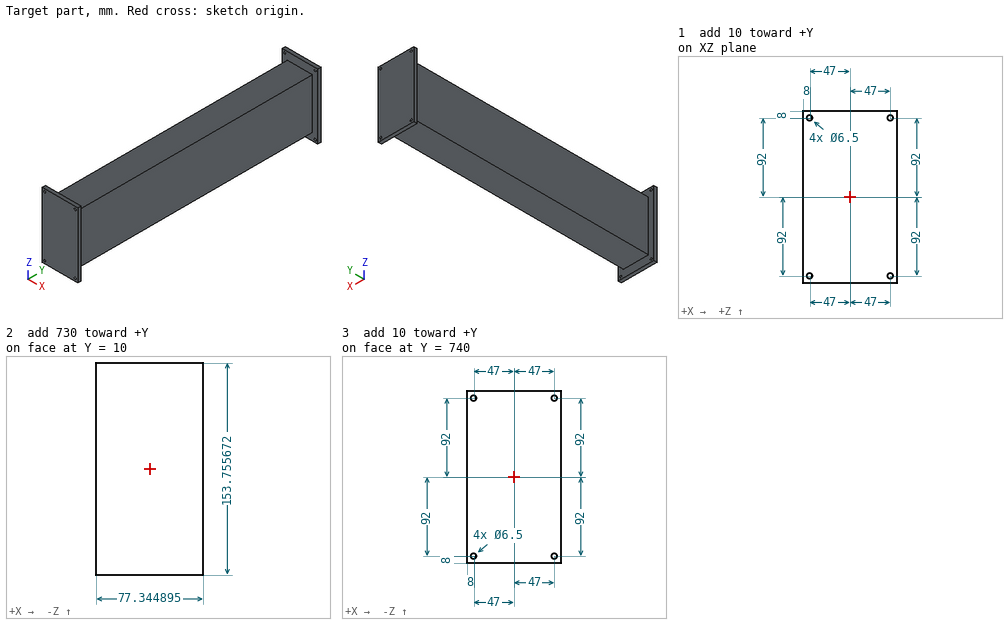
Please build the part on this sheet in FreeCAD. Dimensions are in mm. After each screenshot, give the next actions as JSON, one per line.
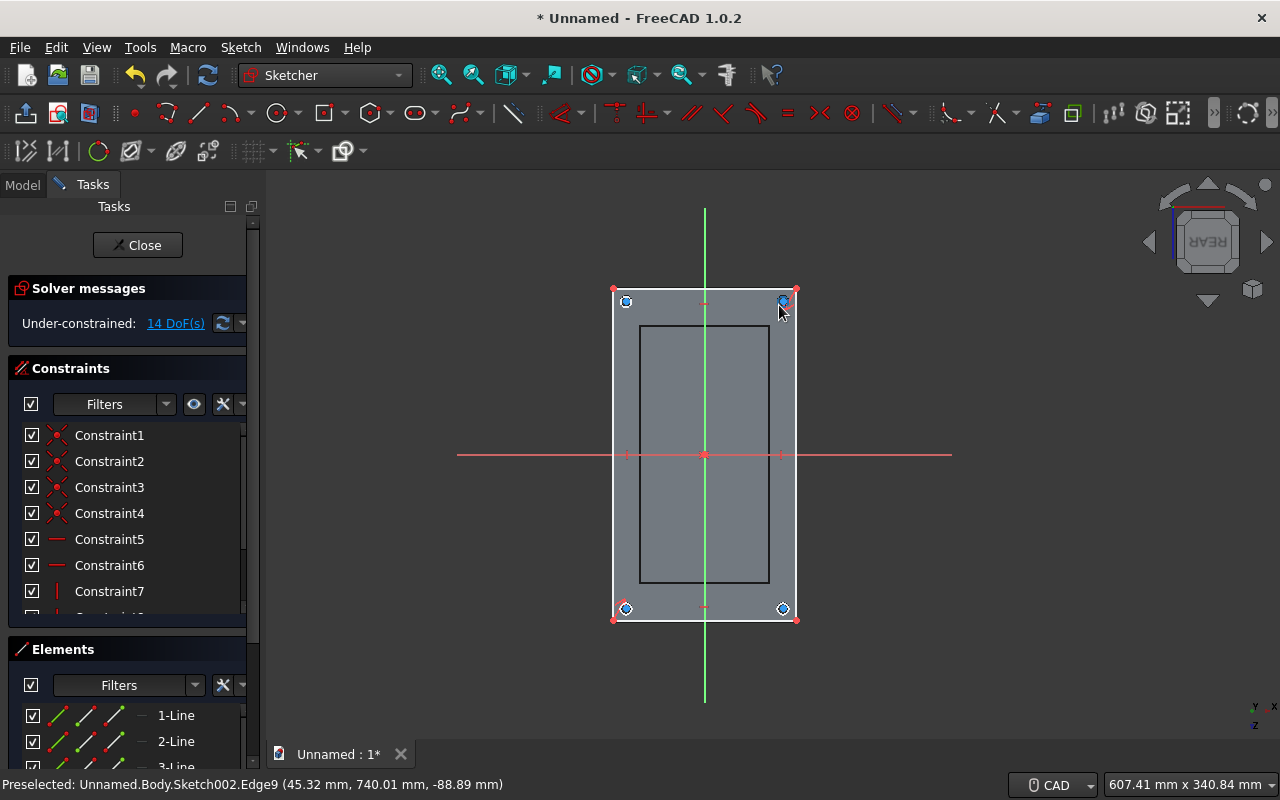
{"action": "scroll", "coordinate": [630, 605], "scroll_direction": "up", "scroll_amount": 5}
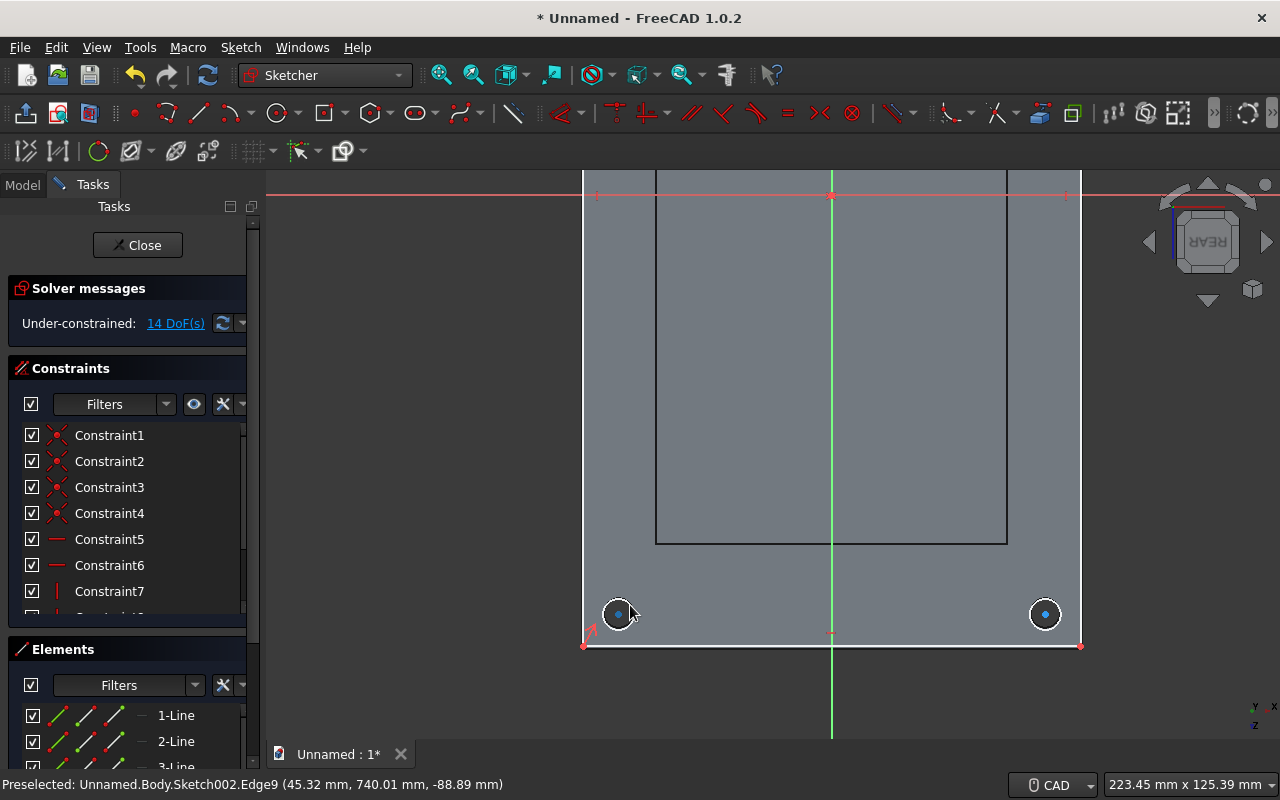
{"action": "left_click", "coordinate": [629, 604]}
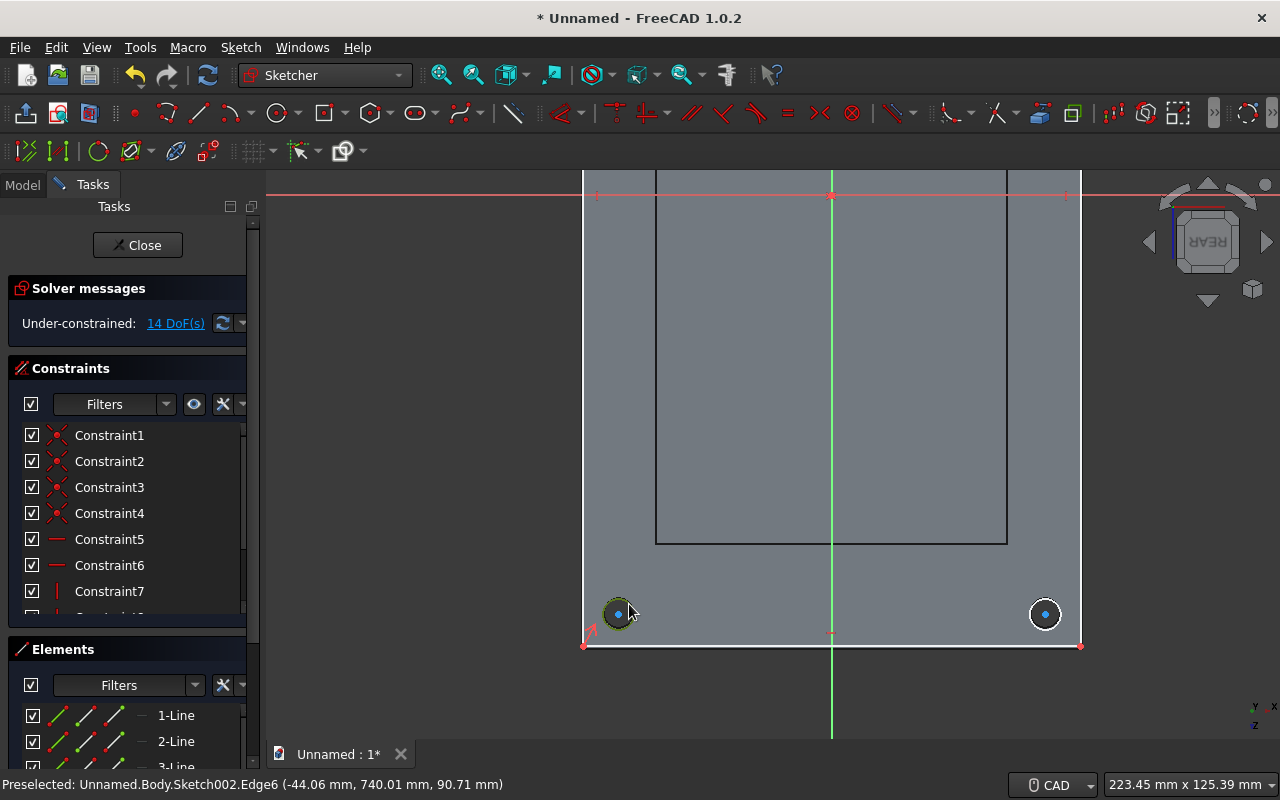
{"action": "left_click", "coordinate": [1056, 604]}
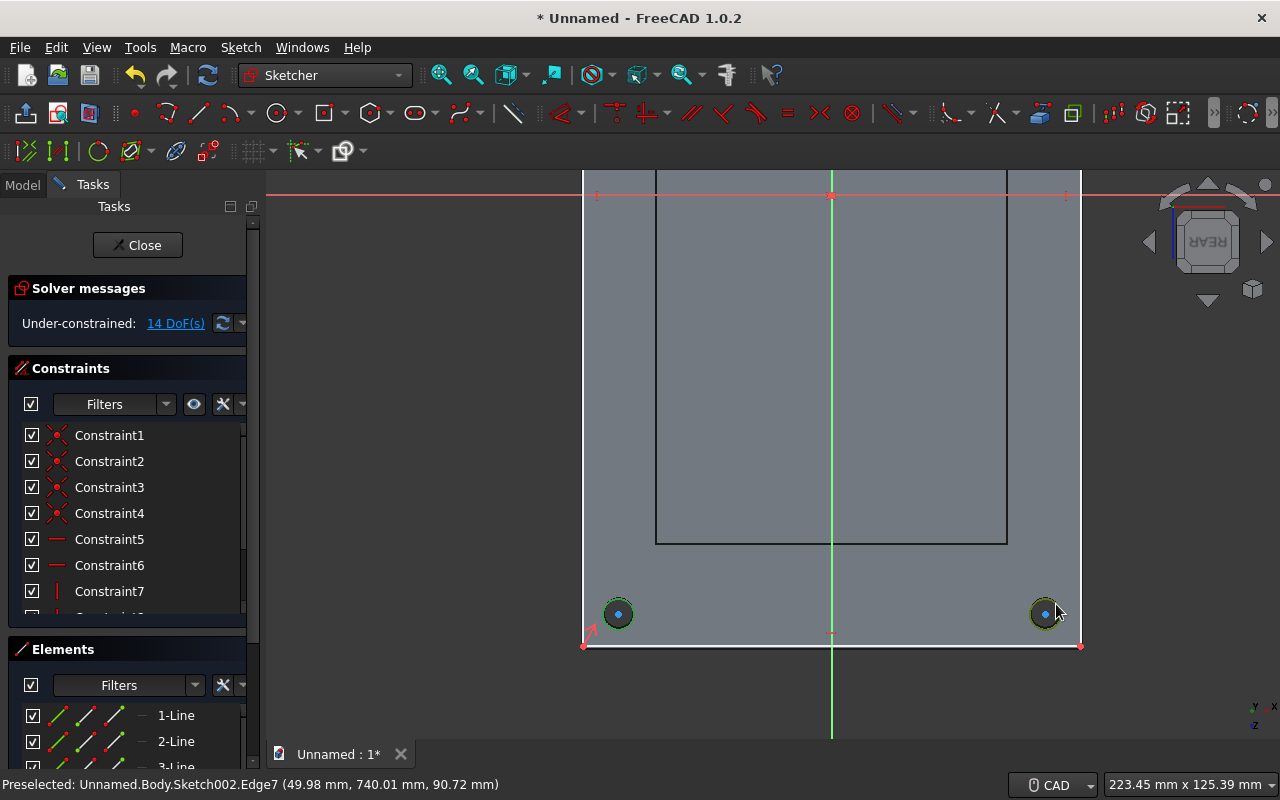
{"action": "scroll", "coordinate": [630, 605], "scroll_direction": "down", "scroll_amount": 5}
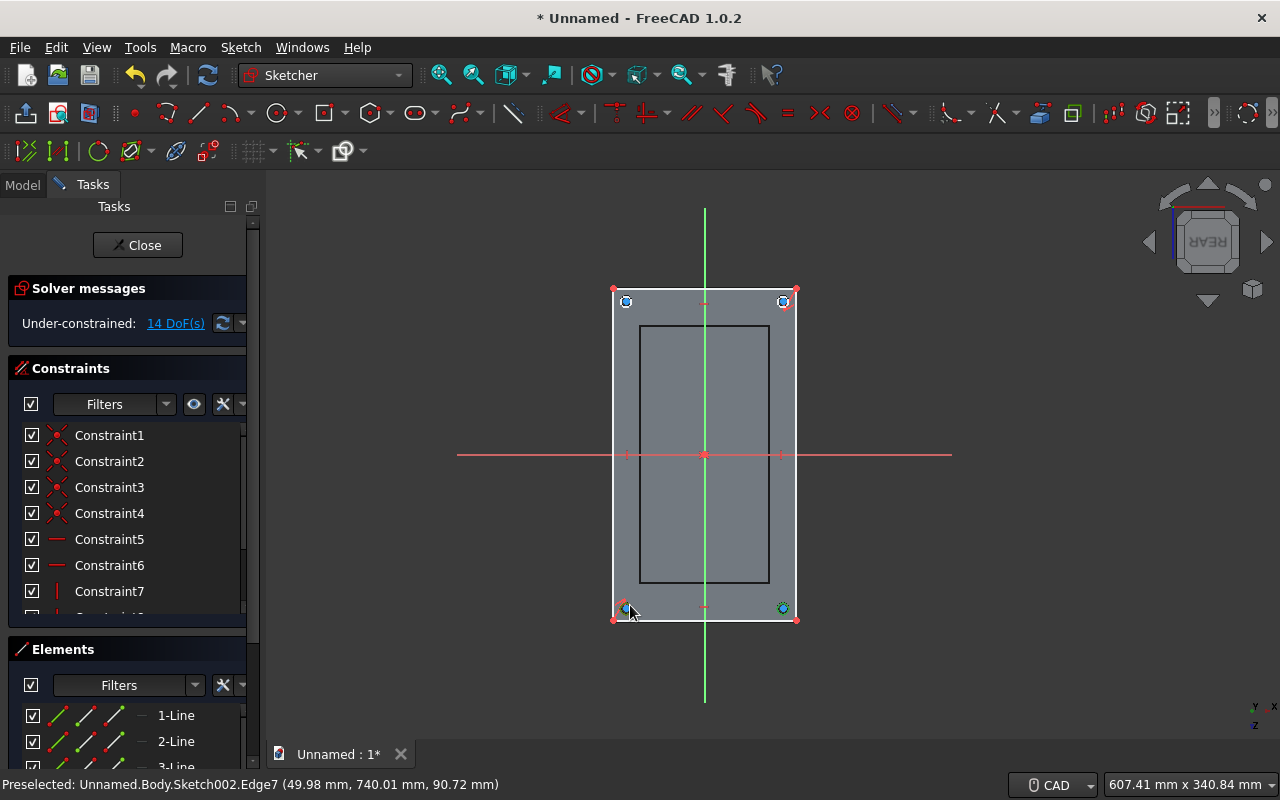
{"action": "scroll", "coordinate": [630, 298], "scroll_direction": "up", "scroll_amount": 5}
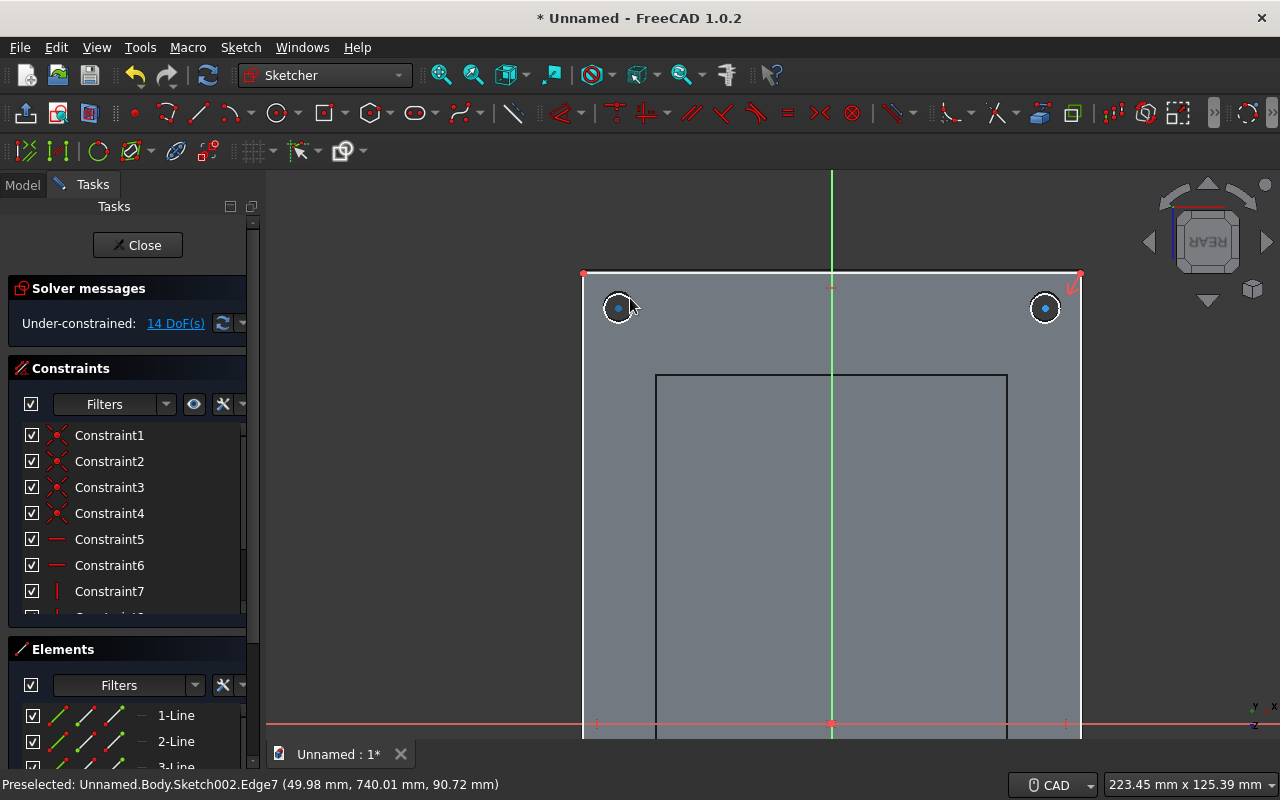
{"action": "left_click", "coordinate": [629, 298]}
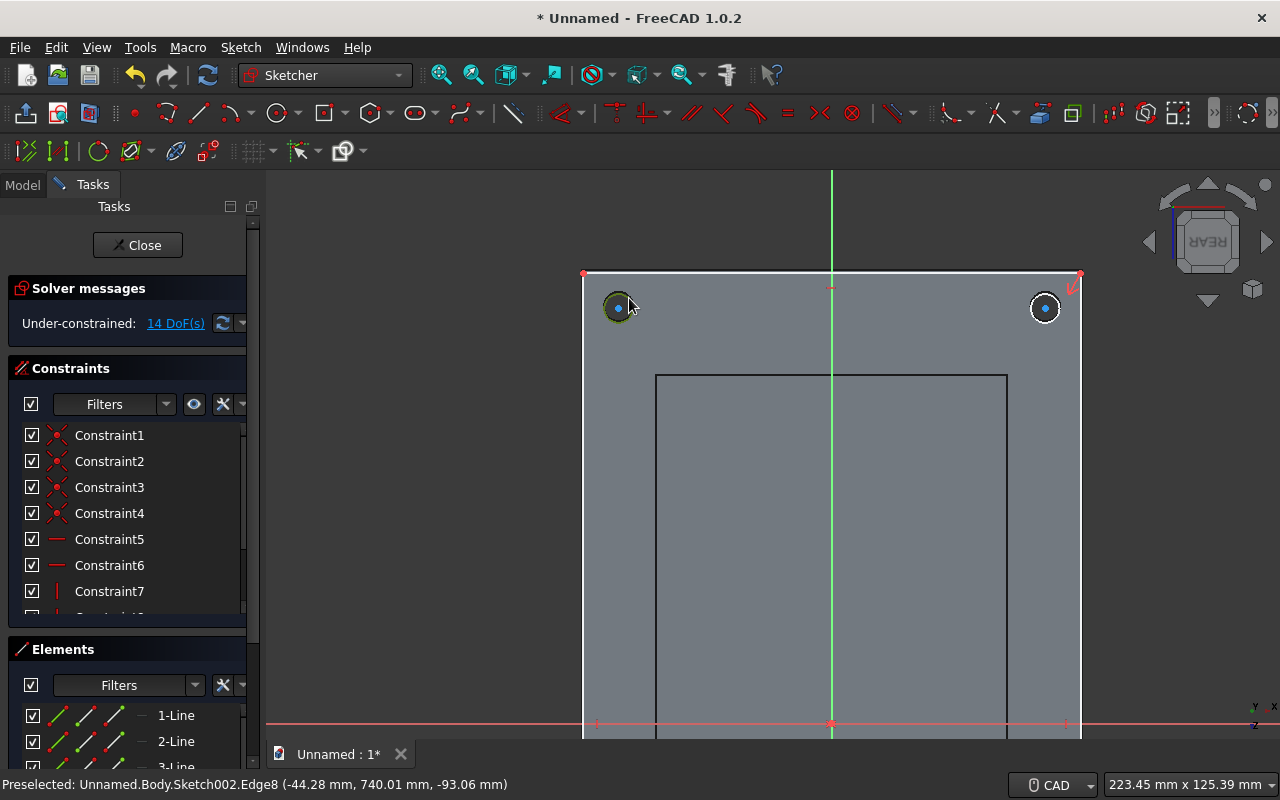
{"action": "left_click", "coordinate": [1055, 298]}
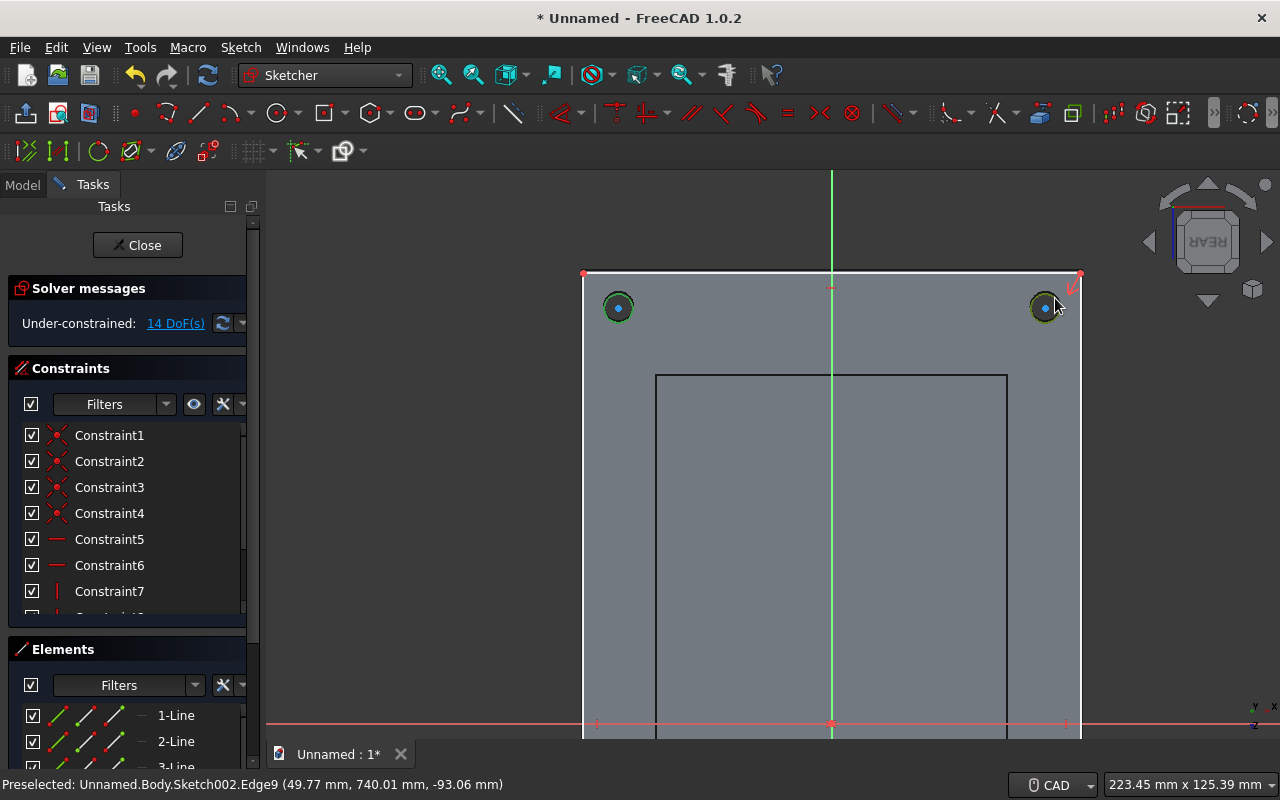
{"action": "left_click", "coordinate": [788, 114]}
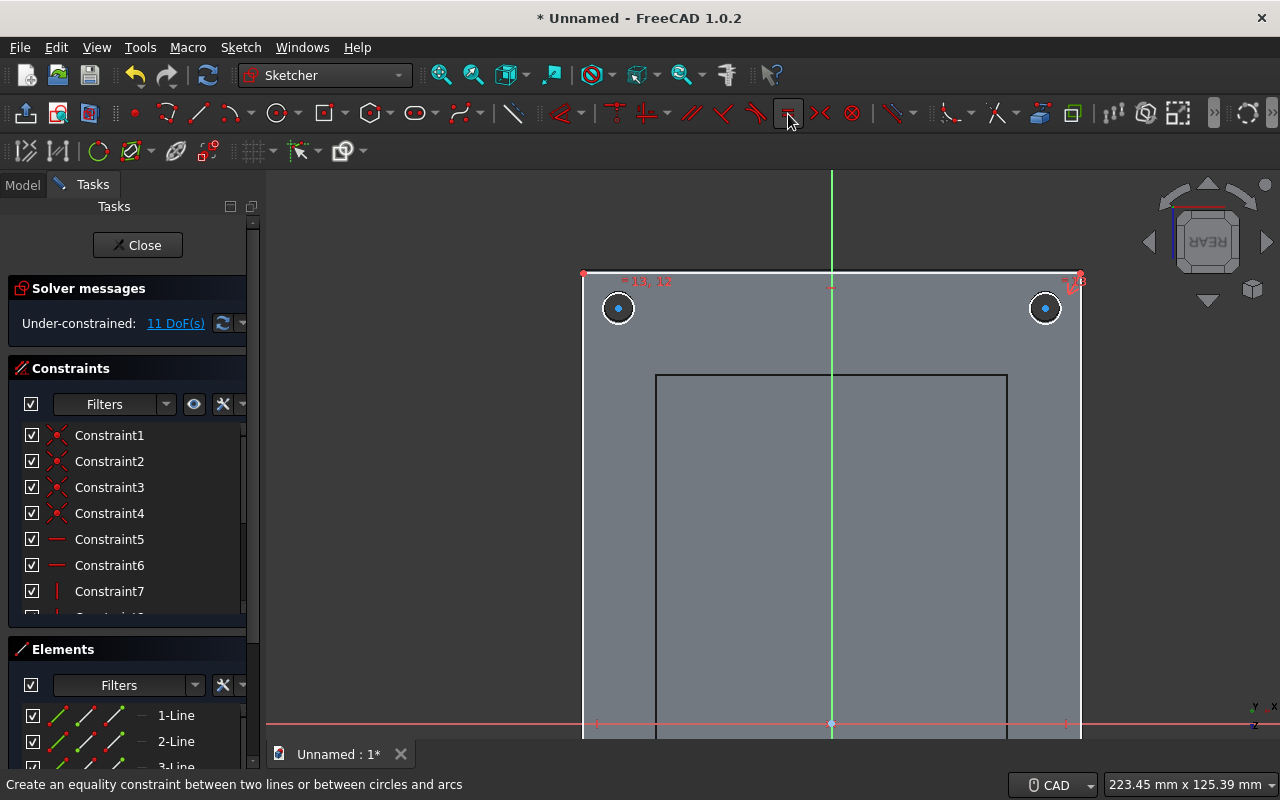
{"action": "left_click", "coordinate": [560, 114]}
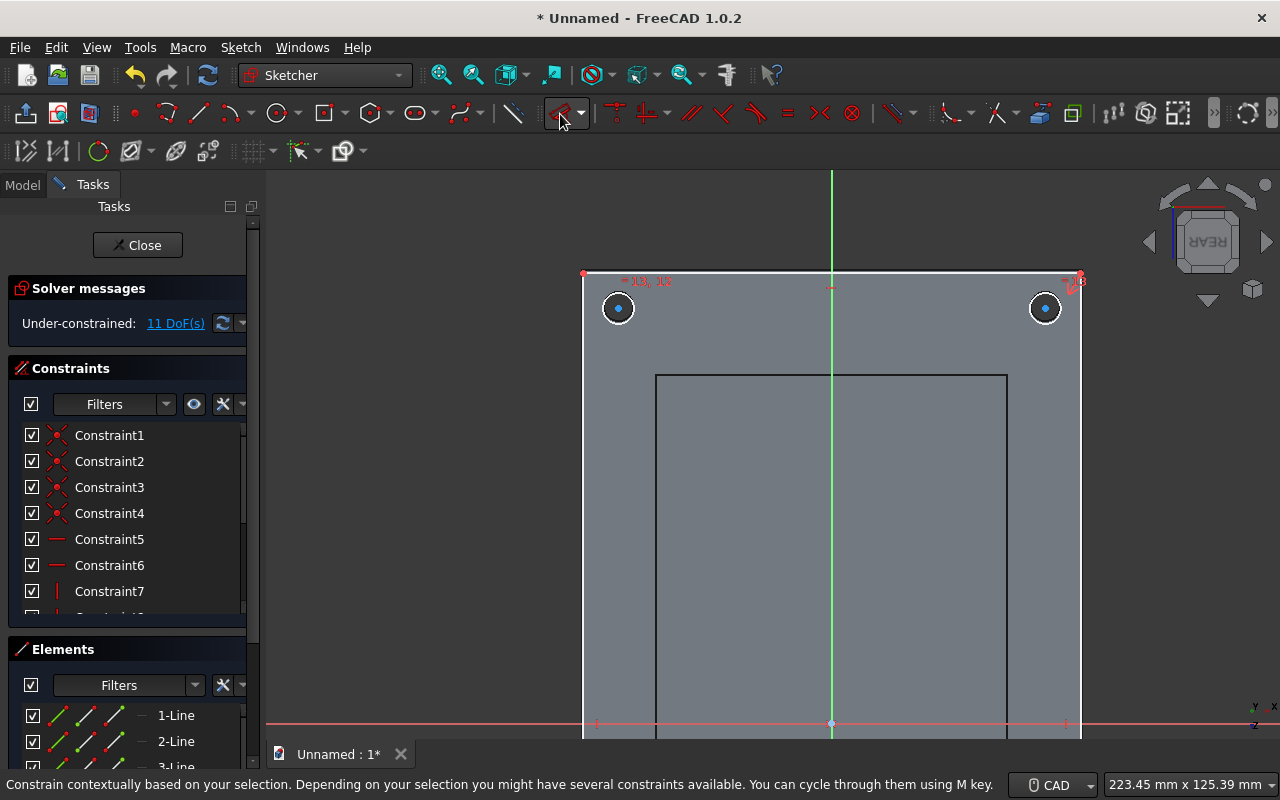
{"action": "scroll", "coordinate": [630, 298], "scroll_direction": "down", "scroll_amount": 5}